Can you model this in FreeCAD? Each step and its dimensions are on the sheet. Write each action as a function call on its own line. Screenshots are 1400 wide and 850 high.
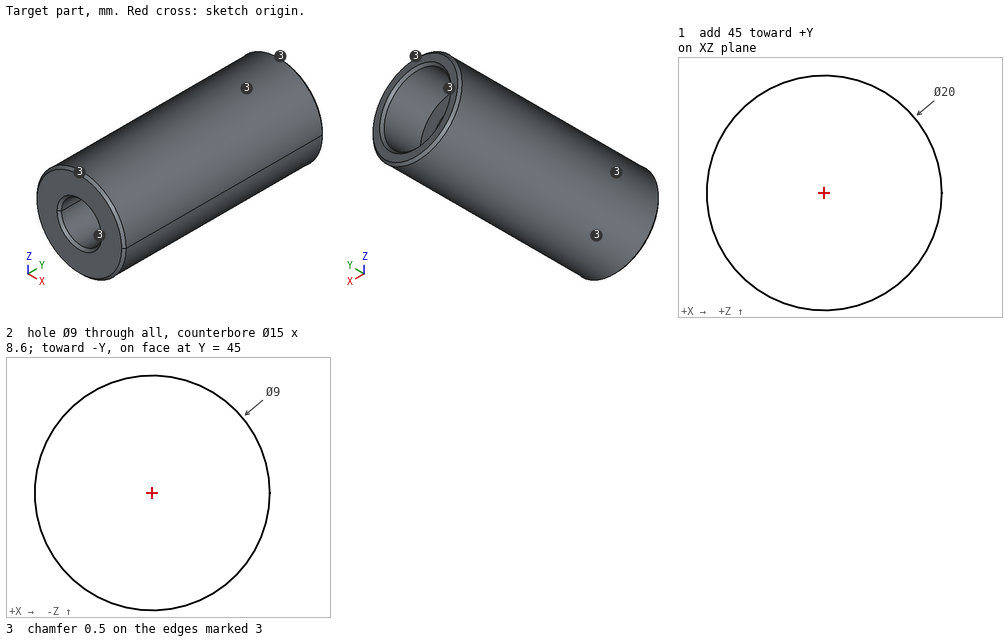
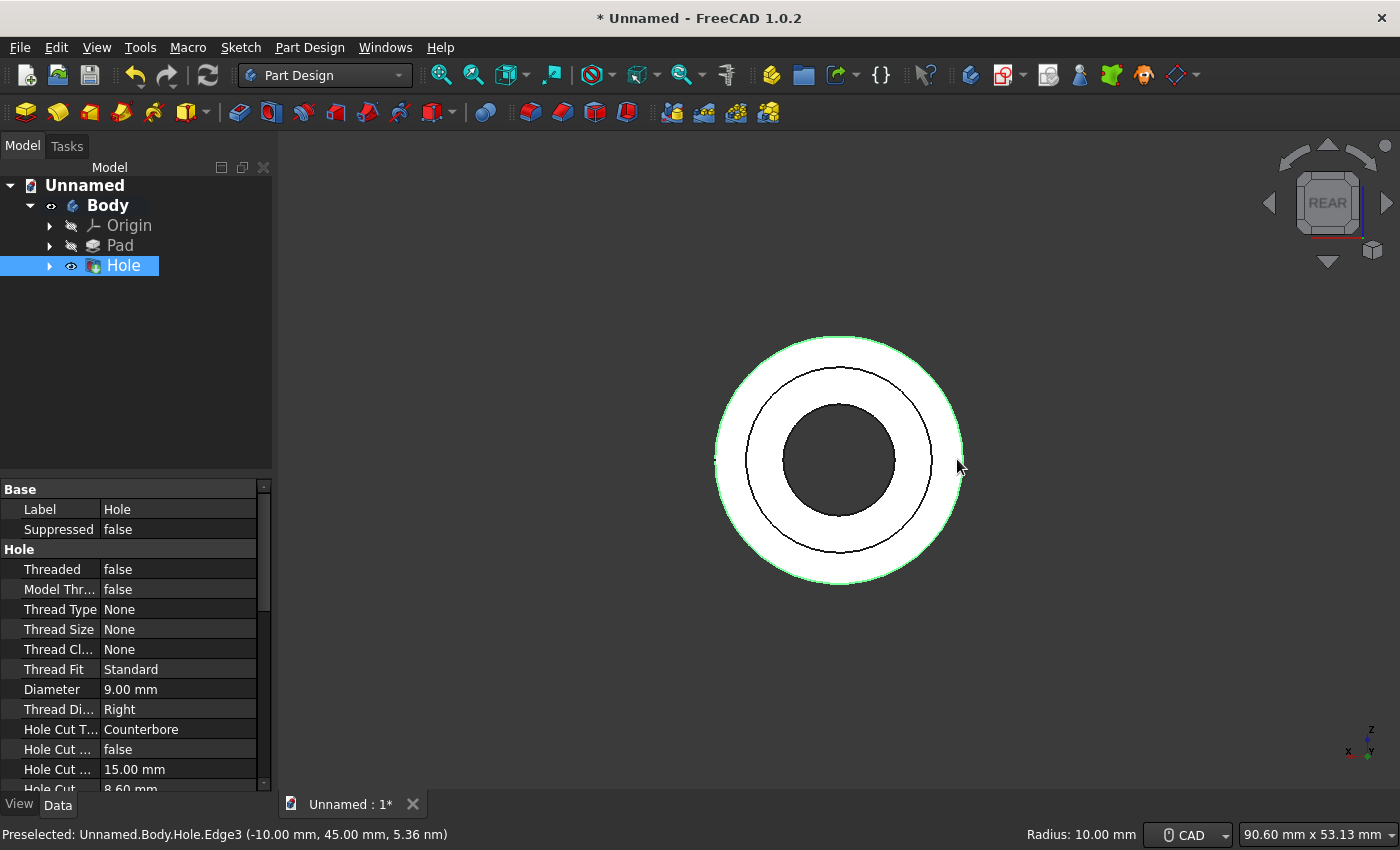
click(746, 459, ctrl)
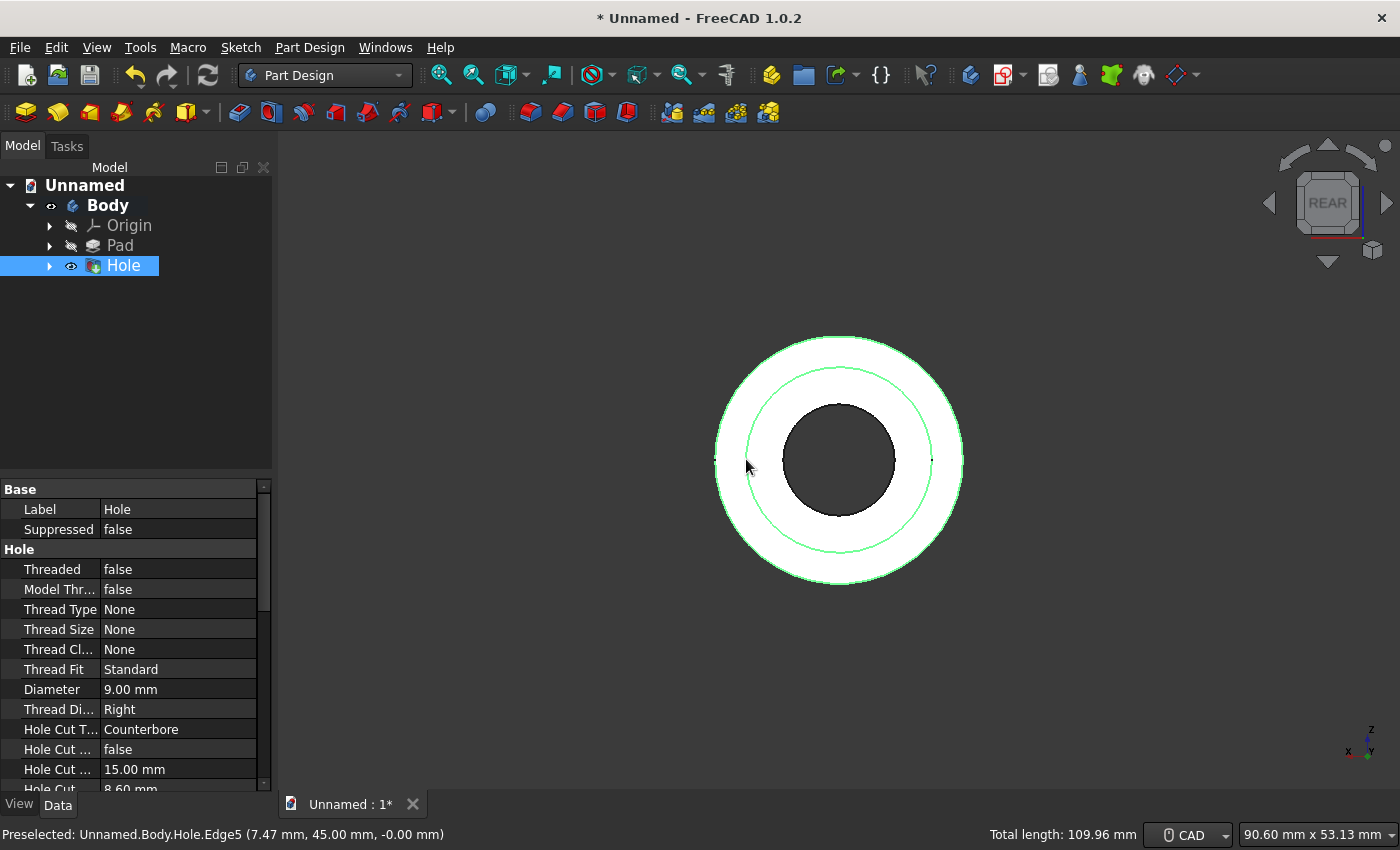
key(0)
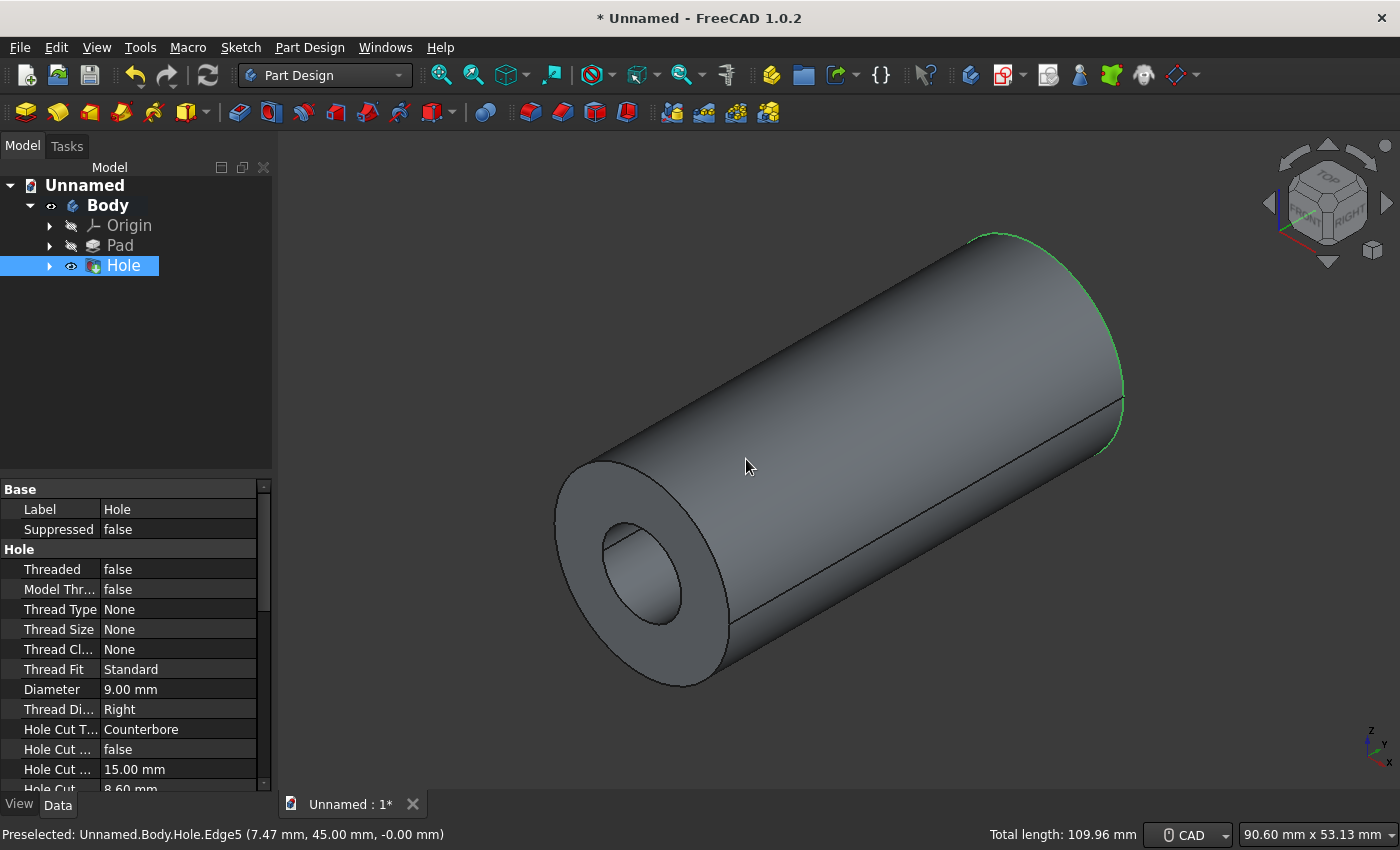
click(615, 461, ctrl)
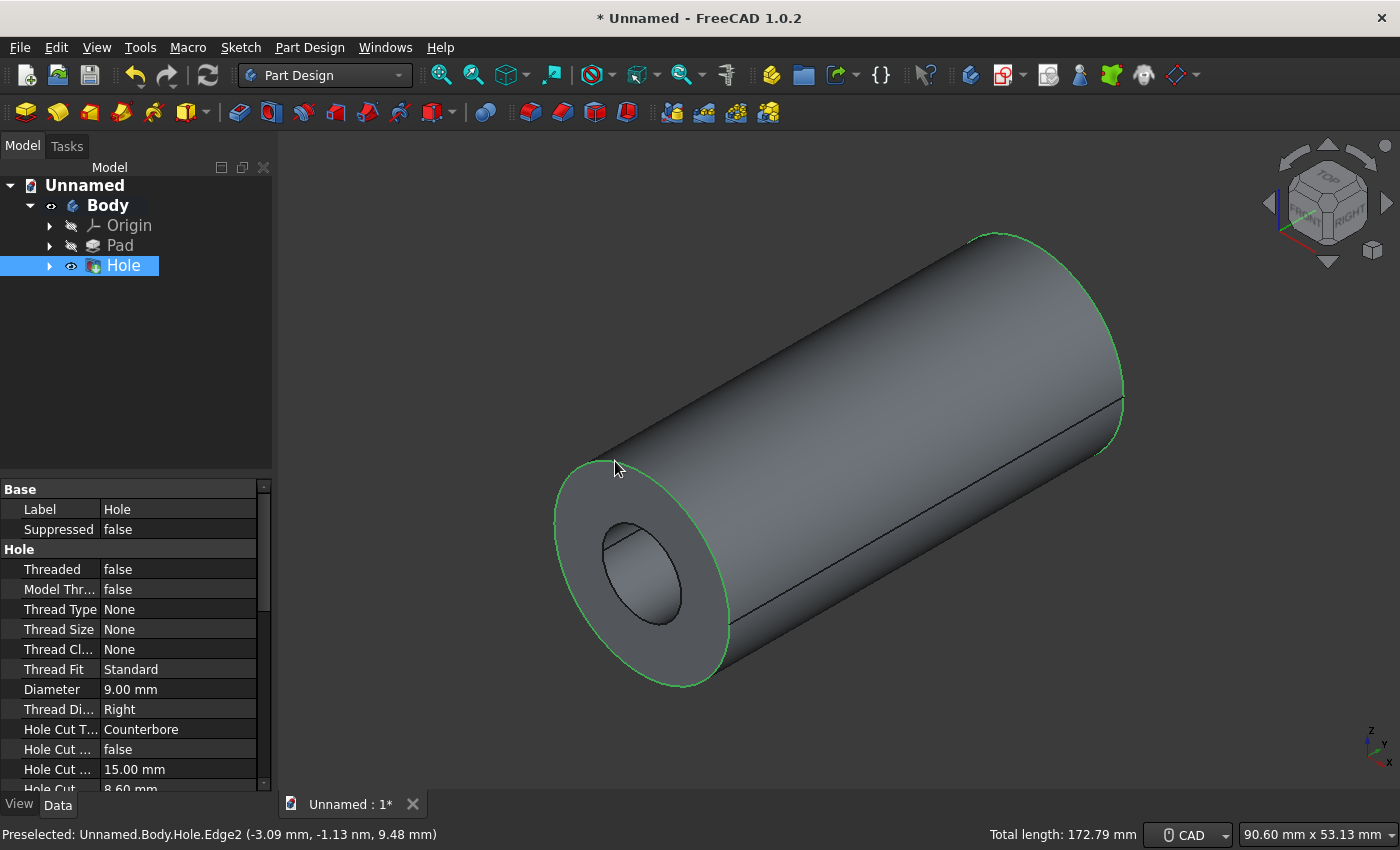
click(654, 623, ctrl)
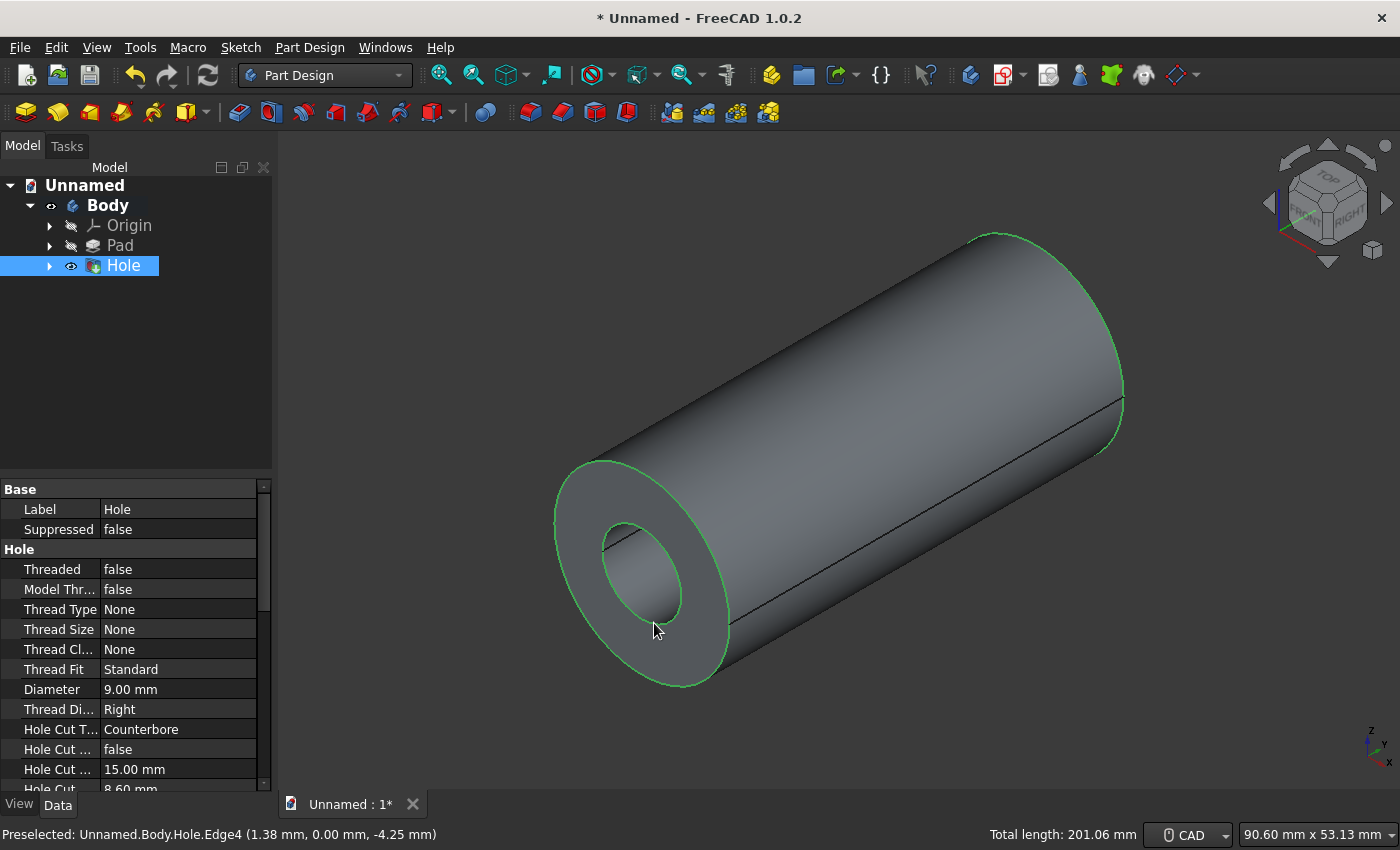
click(564, 112)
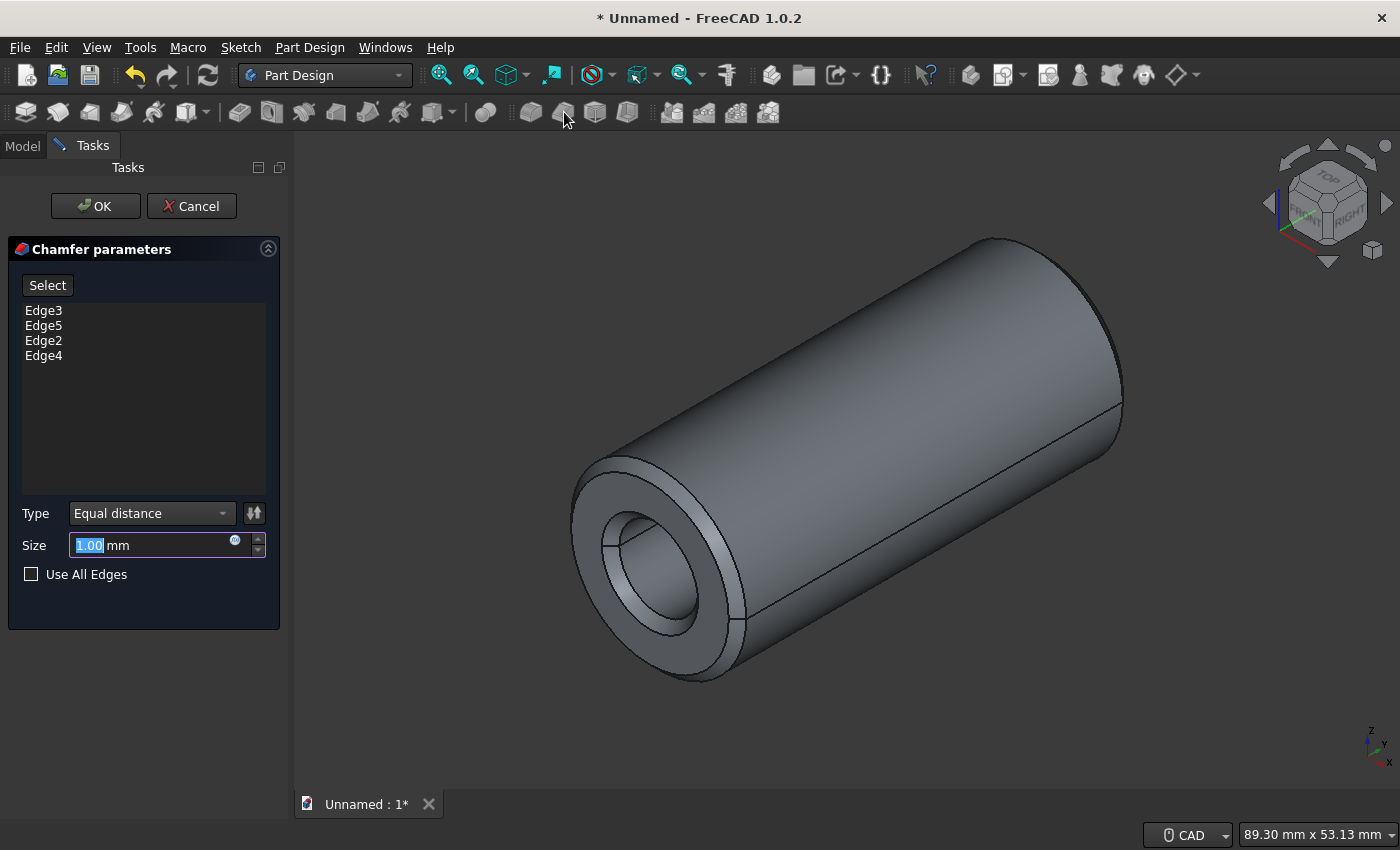
text(0.5)
key(Tab)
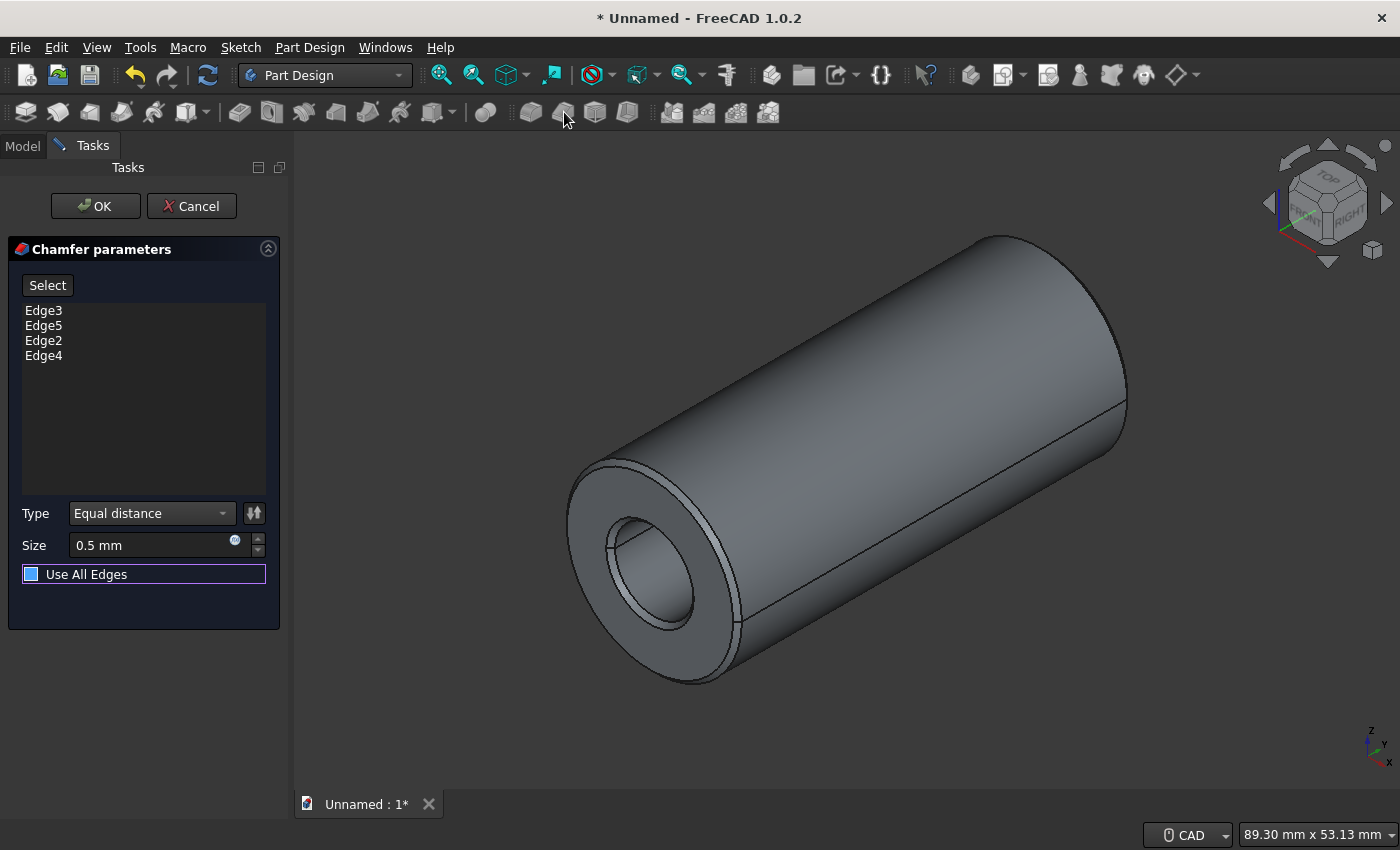
click(96, 206)